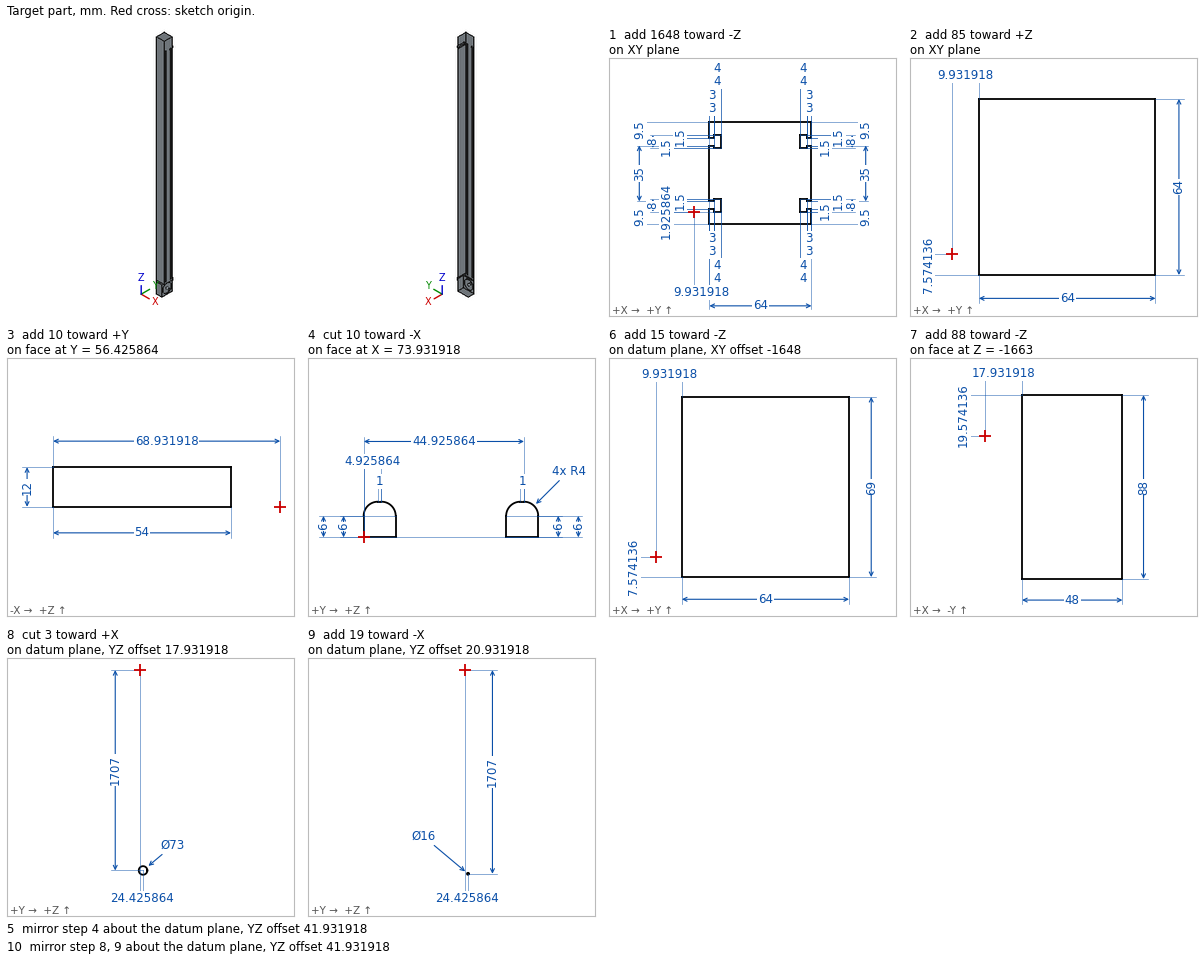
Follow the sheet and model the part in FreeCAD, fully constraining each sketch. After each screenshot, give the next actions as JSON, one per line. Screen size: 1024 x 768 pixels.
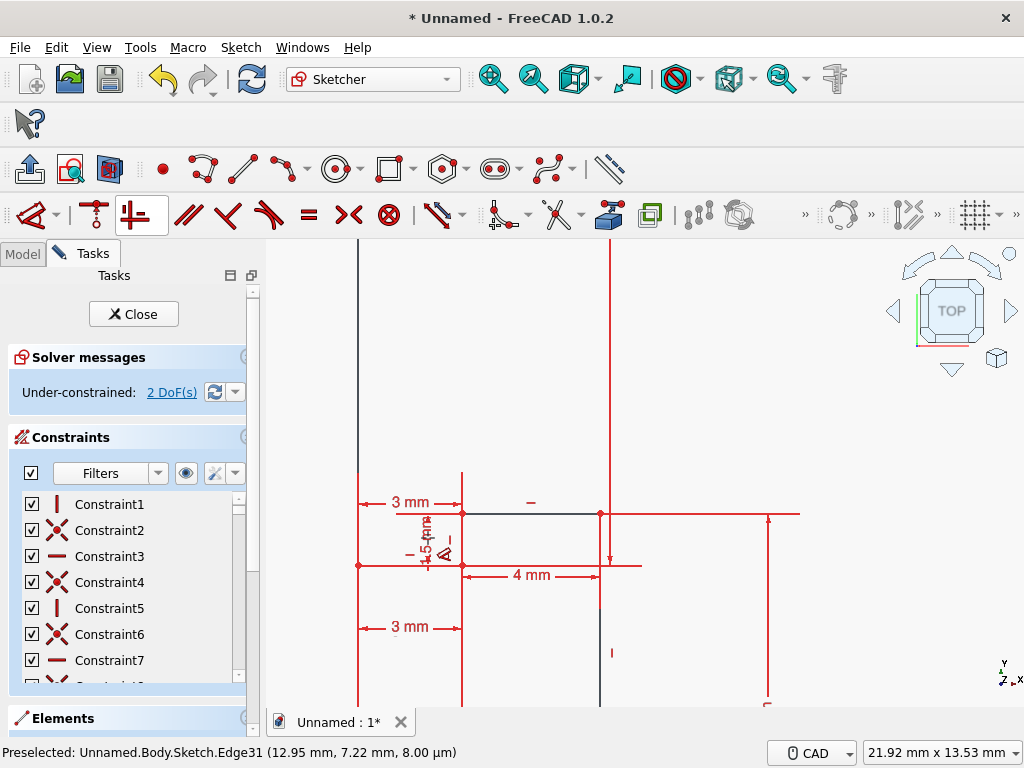
{"action": "scroll", "coordinate": [464, 554], "scroll_direction": "down", "scroll_amount": 10}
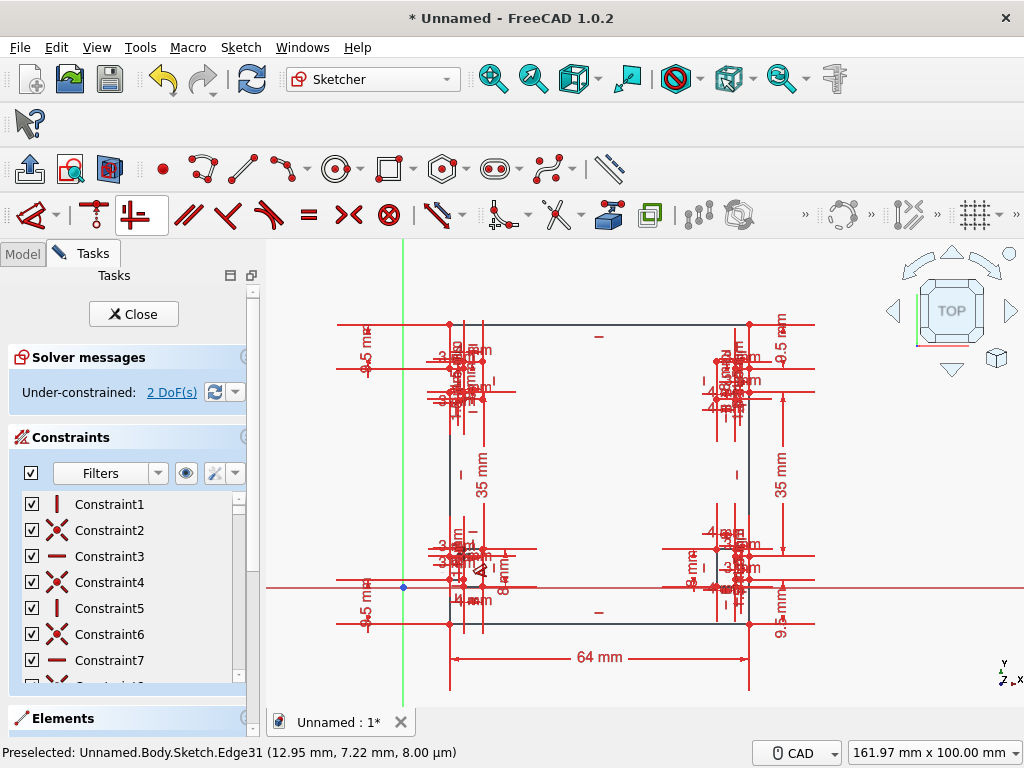
{"action": "left_click", "coordinate": [450, 580]}
{"action": "left_click", "coordinate": [427, 622]}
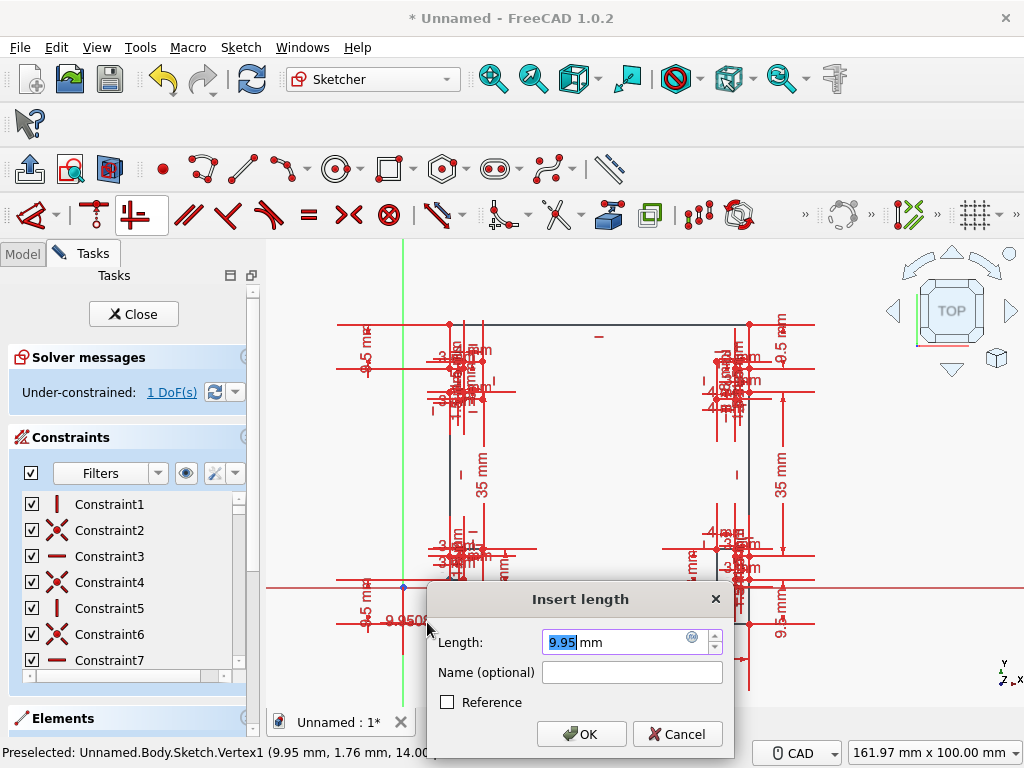
{"action": "type", "text": "9.931918"}
{"action": "key", "text": "Return"}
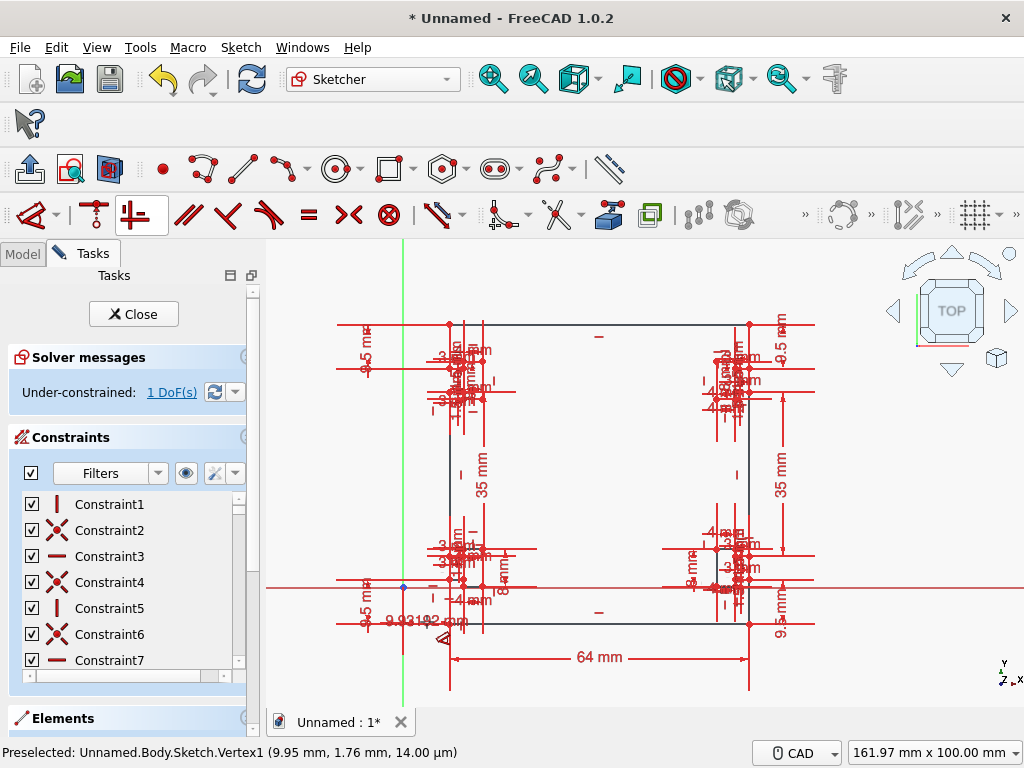
{"action": "scroll", "coordinate": [450, 580], "scroll_direction": "up", "scroll_amount": 8}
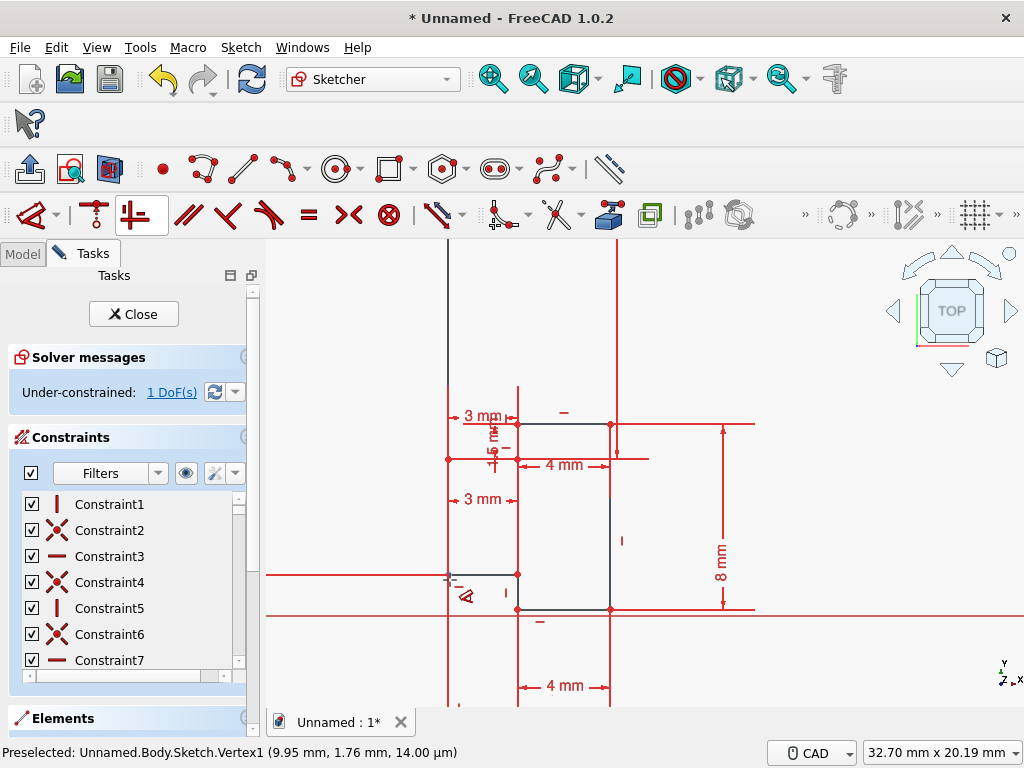
{"action": "left_click", "coordinate": [448, 575]}
{"action": "left_click", "coordinate": [482, 595]}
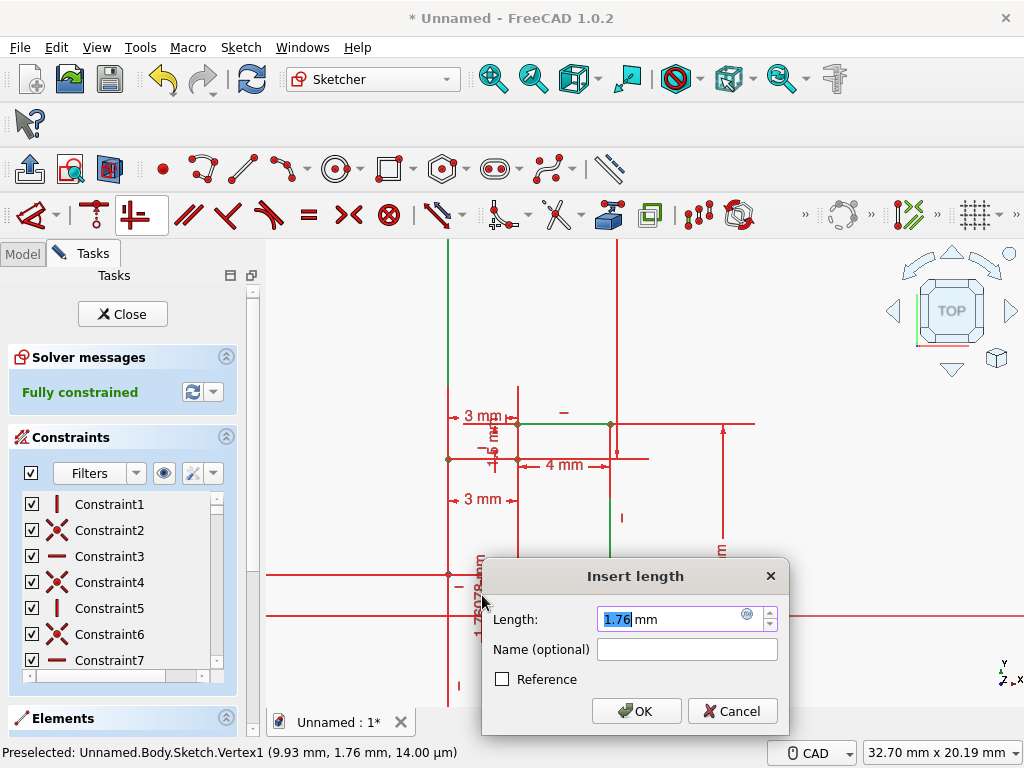
{"action": "type", "text": "1.925864"}
{"action": "key", "text": "Return"}
{"action": "key", "text": "Escape"}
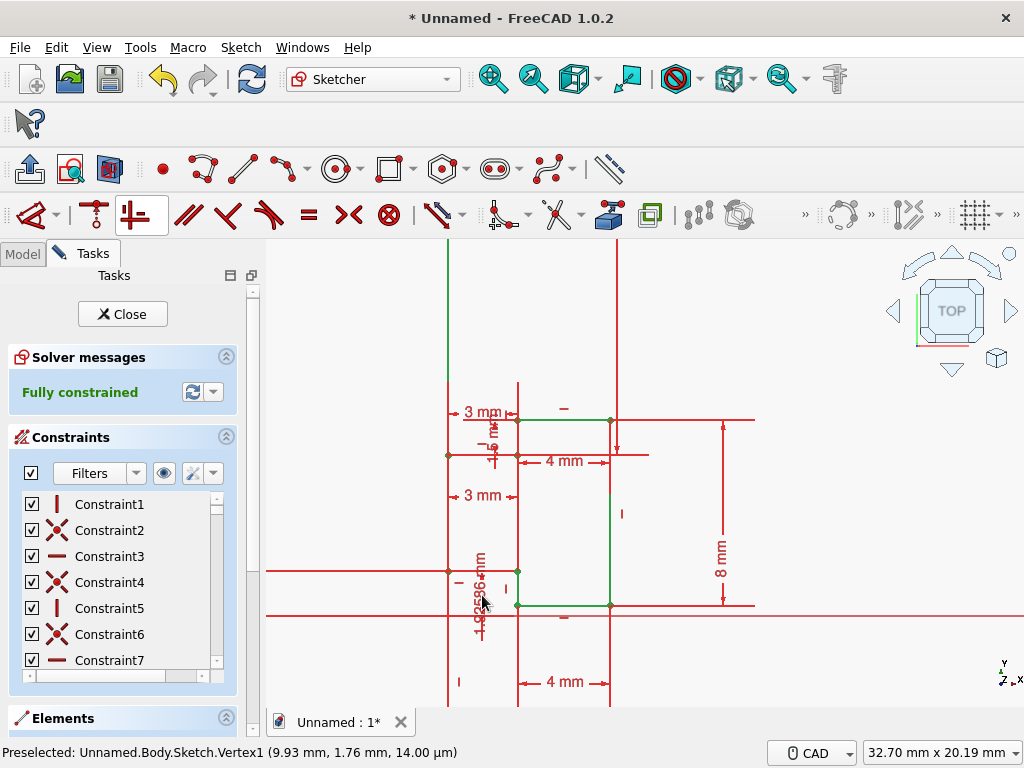
{"action": "left_click", "coordinate": [123, 314]}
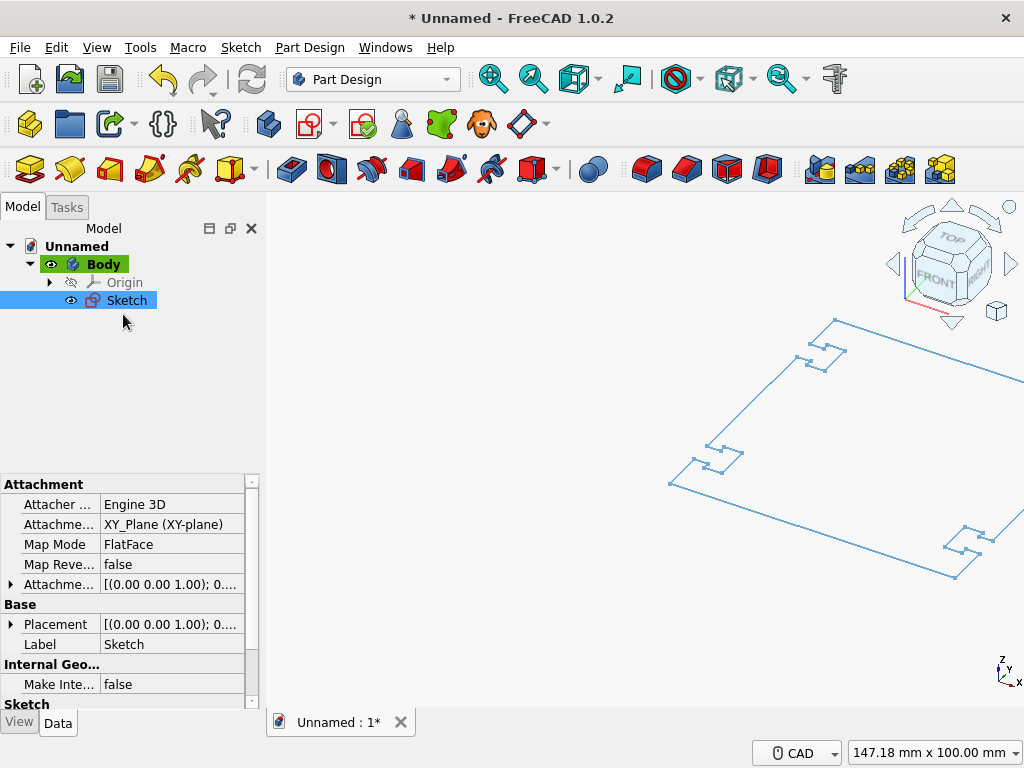
{"action": "left_click", "coordinate": [30, 170]}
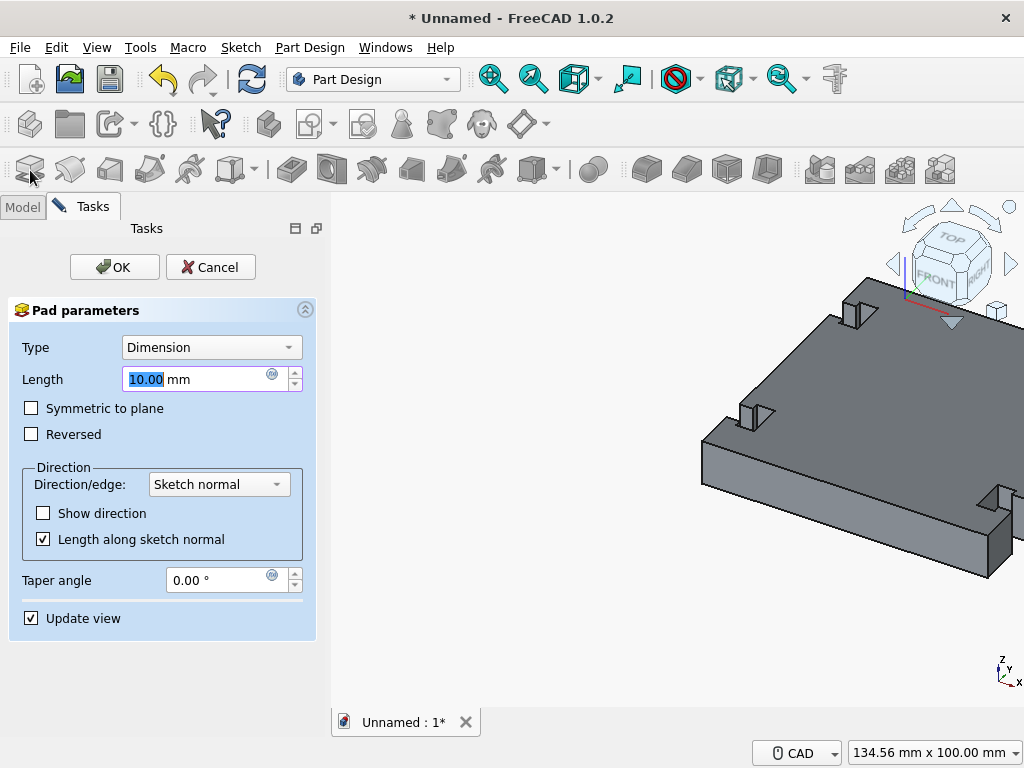
{"action": "type", "text": "1648"}
{"action": "key", "text": "Tab"}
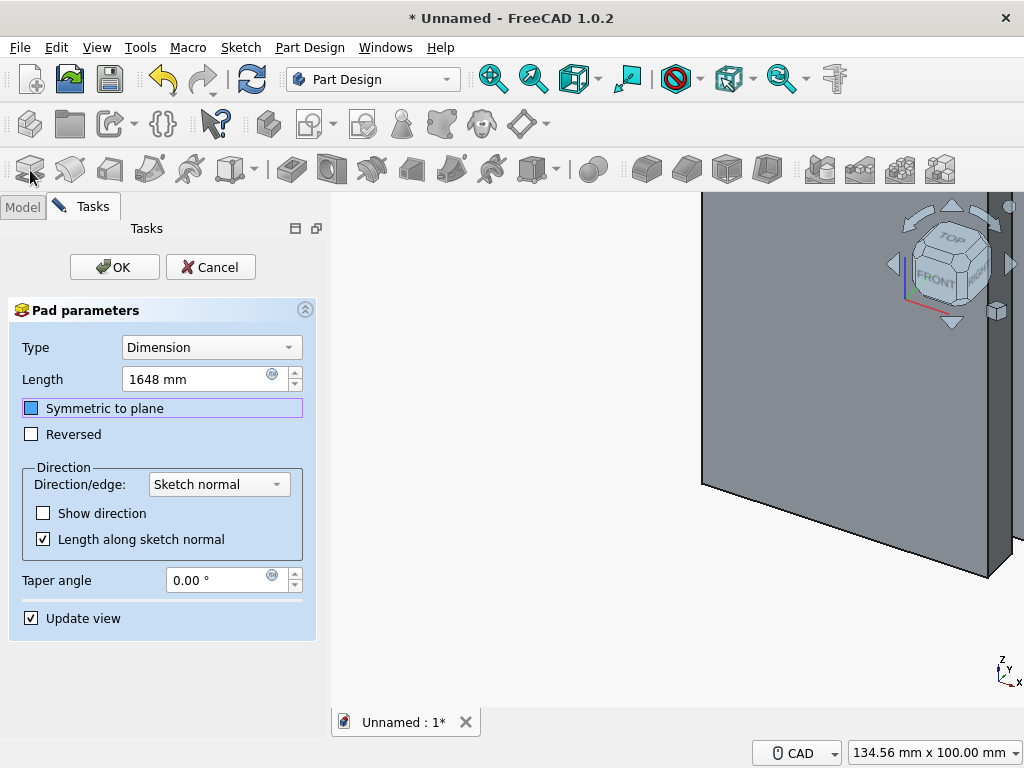
{"action": "left_click", "coordinate": [30, 434]}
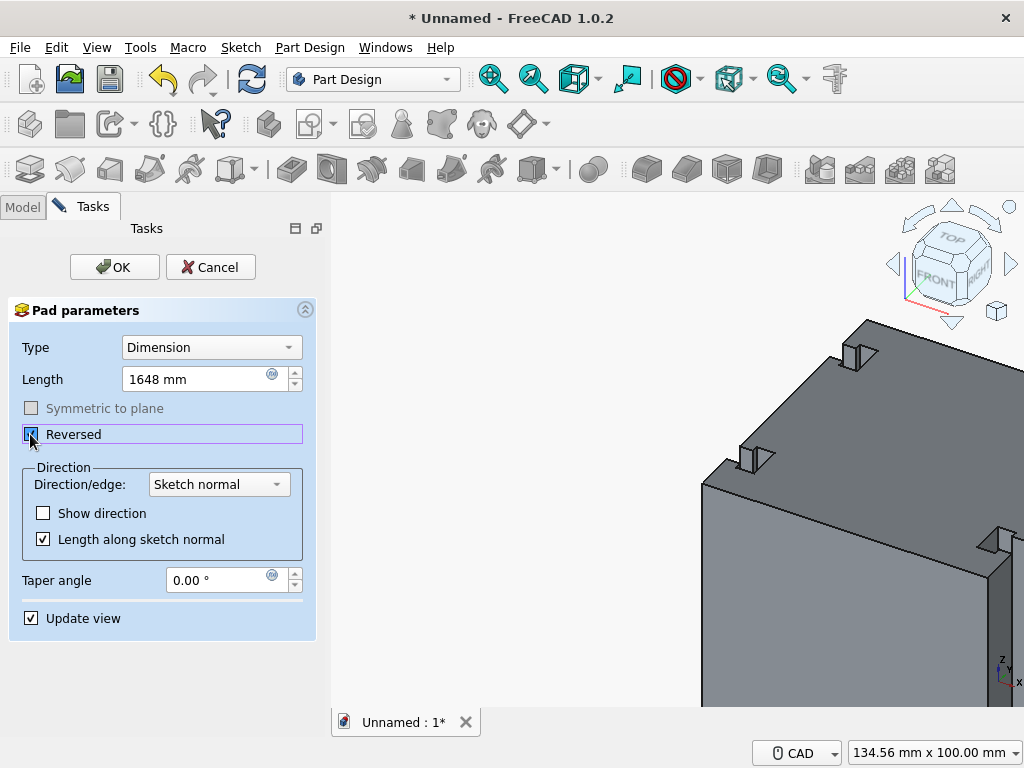
{"action": "left_click", "coordinate": [115, 267]}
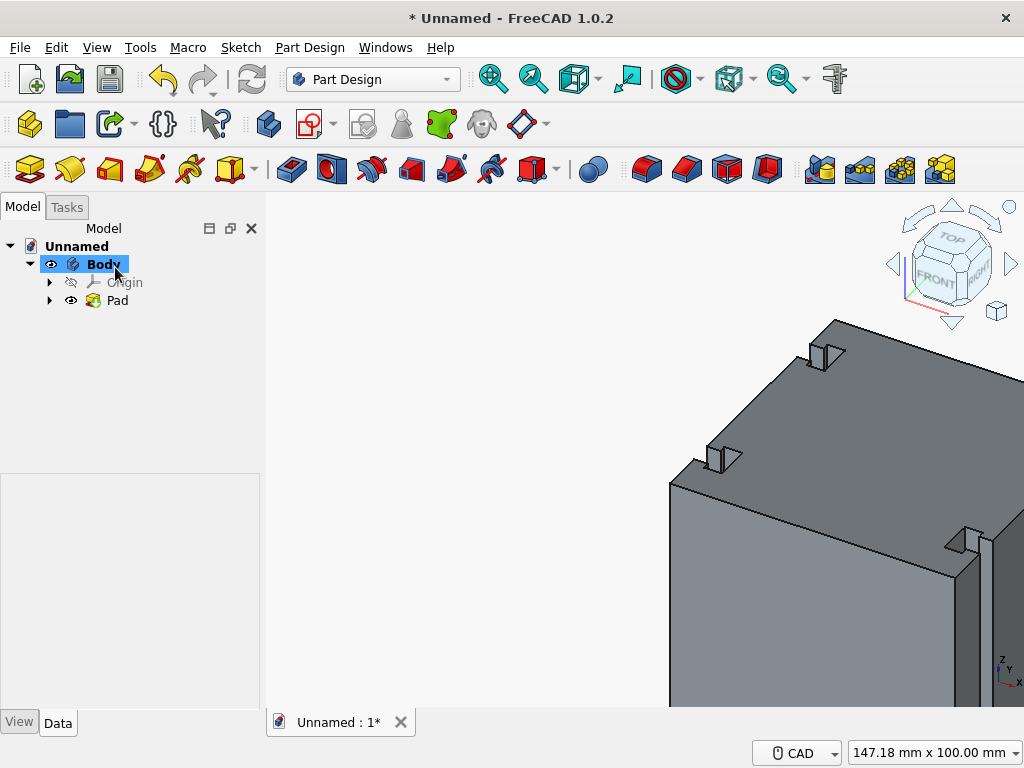
{"action": "left_click", "coordinate": [494, 80]}